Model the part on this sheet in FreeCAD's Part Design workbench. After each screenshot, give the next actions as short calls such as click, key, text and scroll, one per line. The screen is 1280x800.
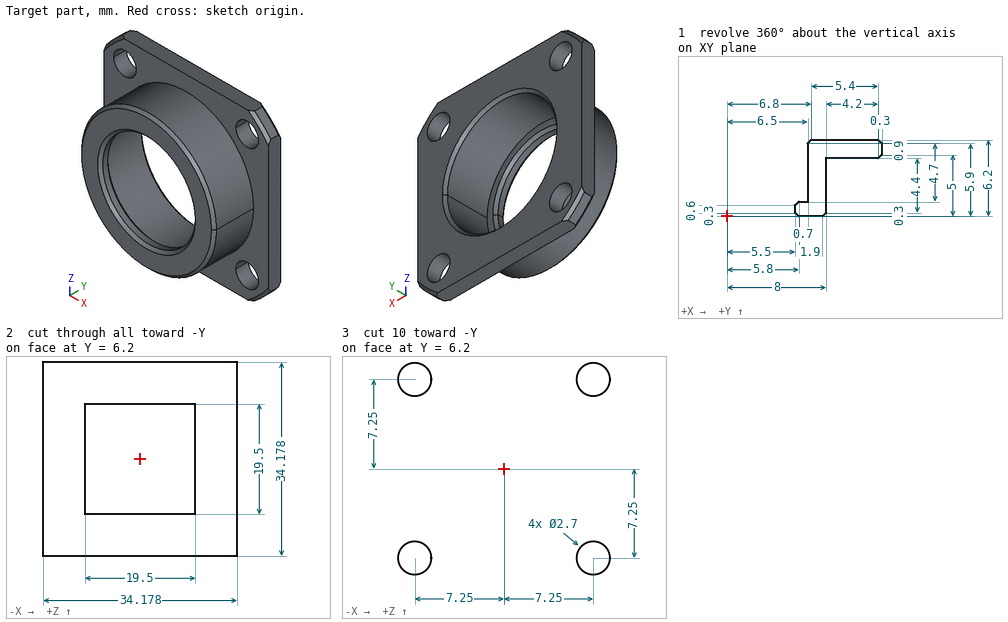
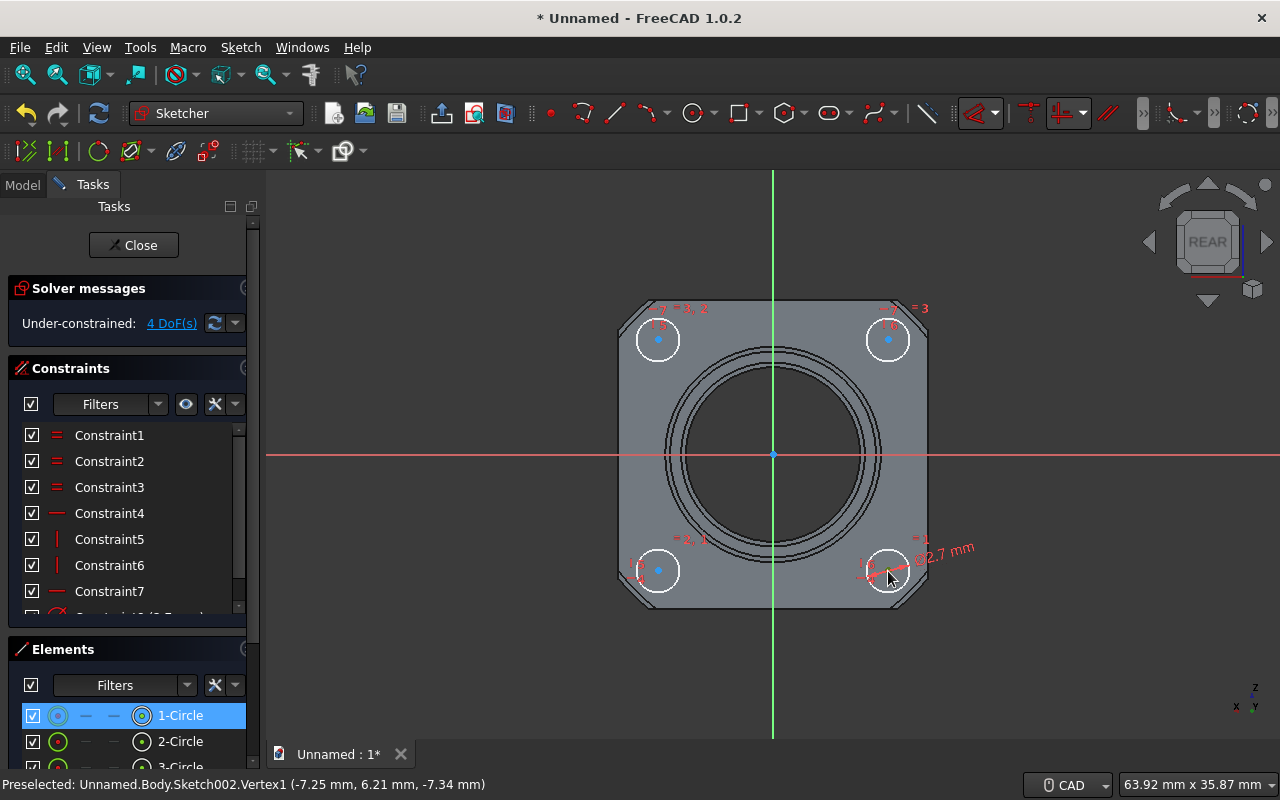
click(998, 114)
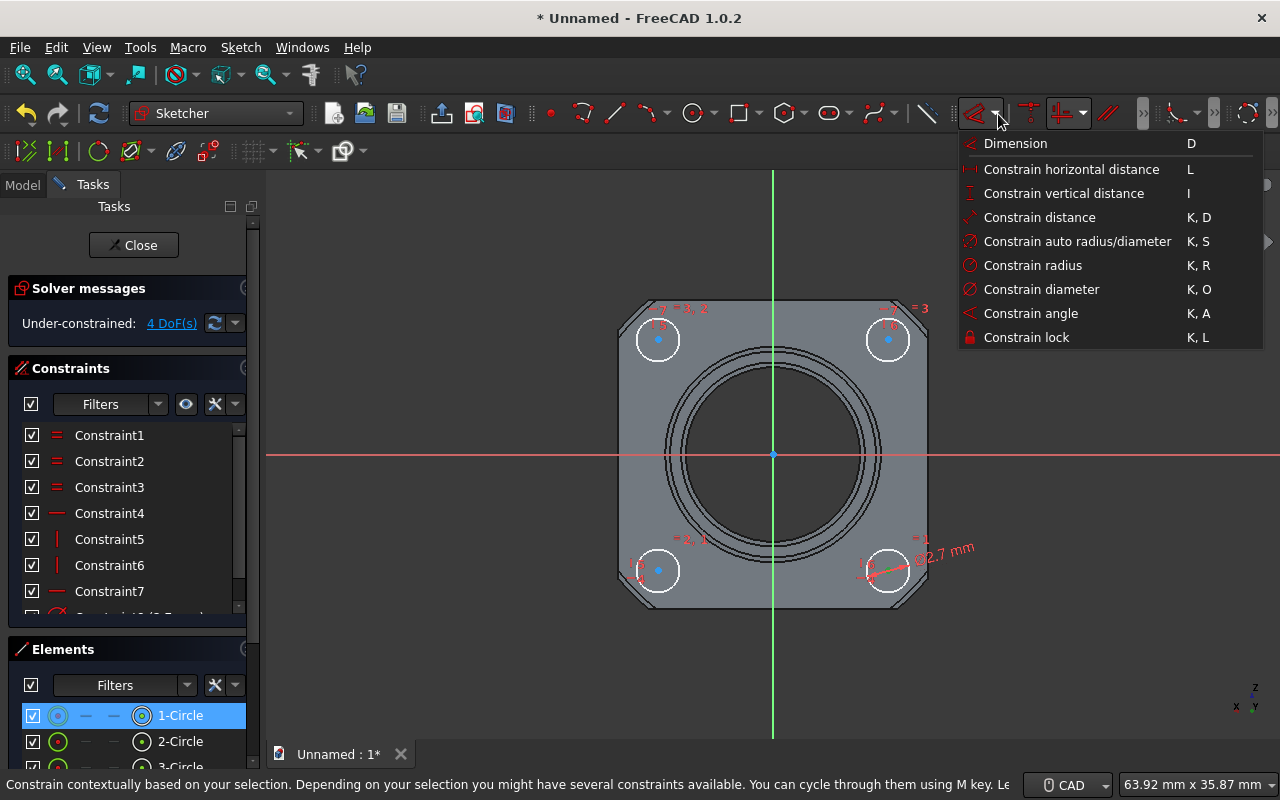
click(1111, 169)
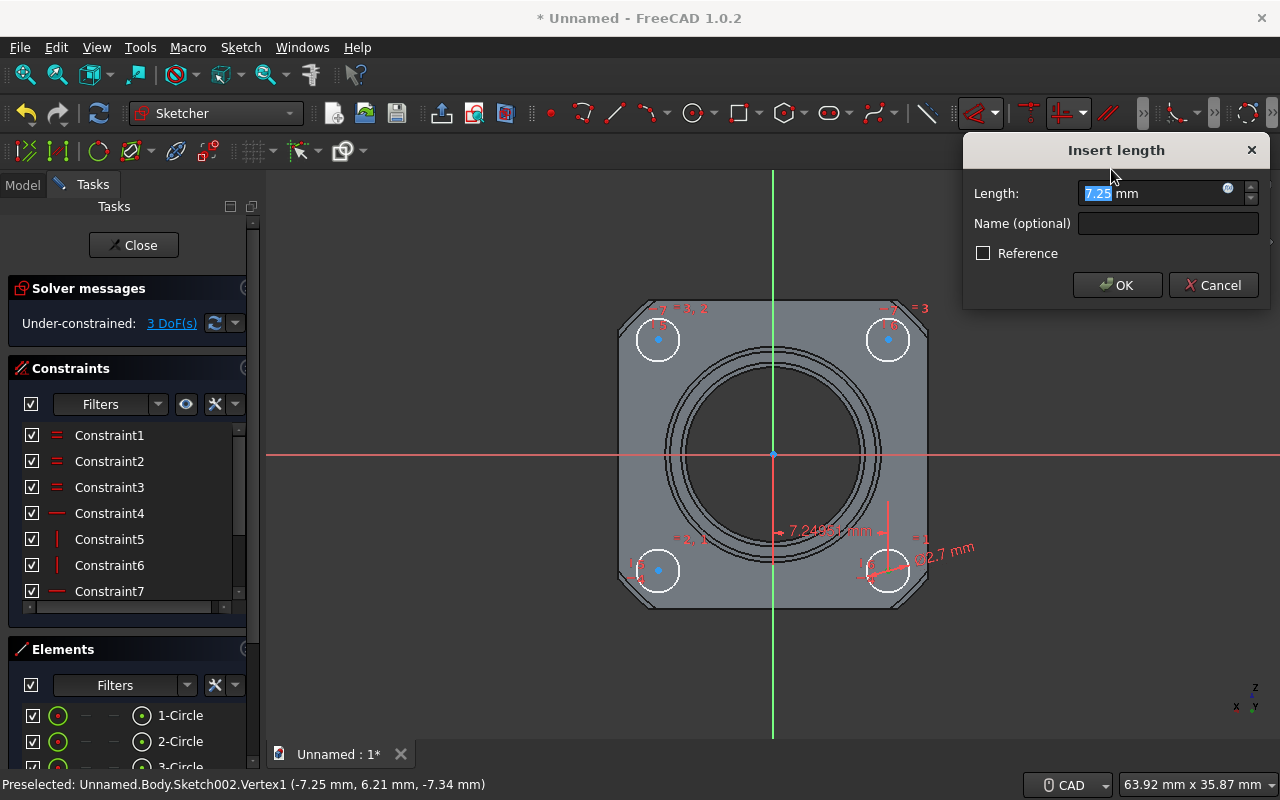
text(7.25)
key(Return)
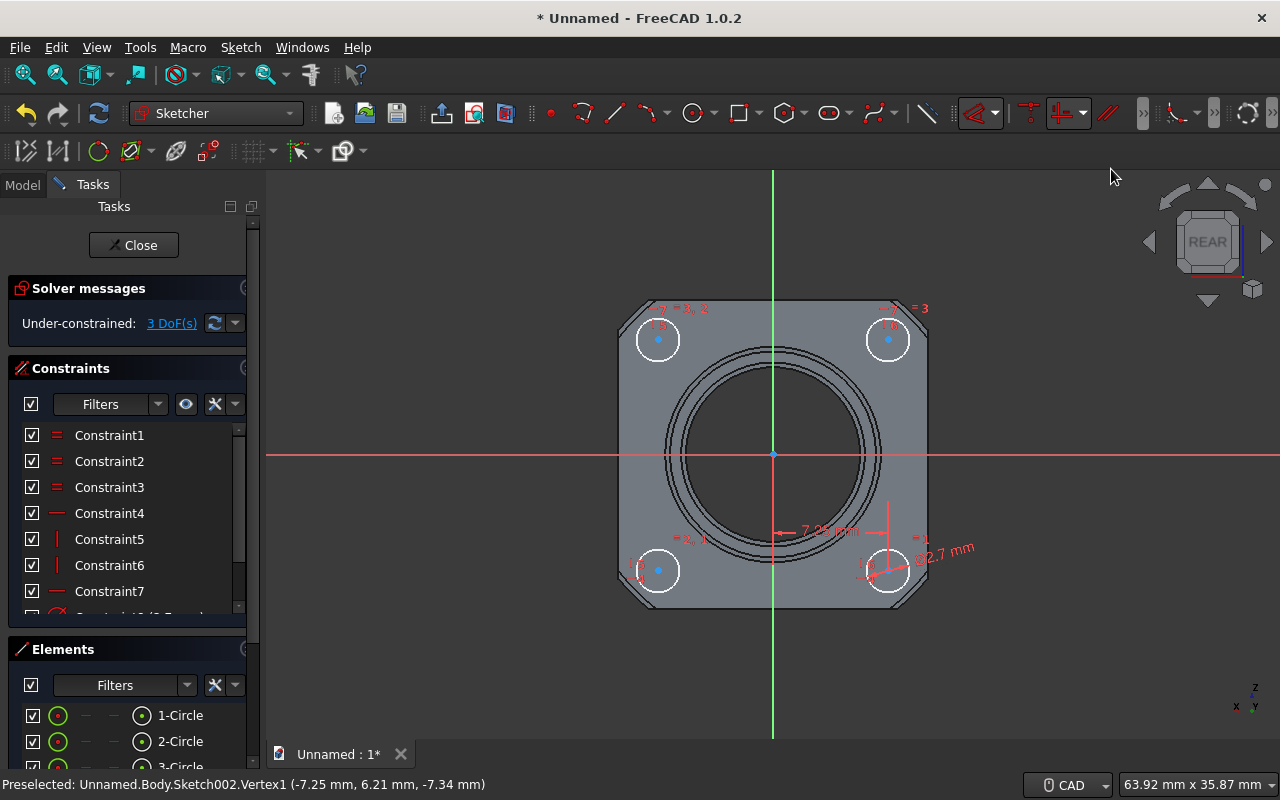
click(888, 571)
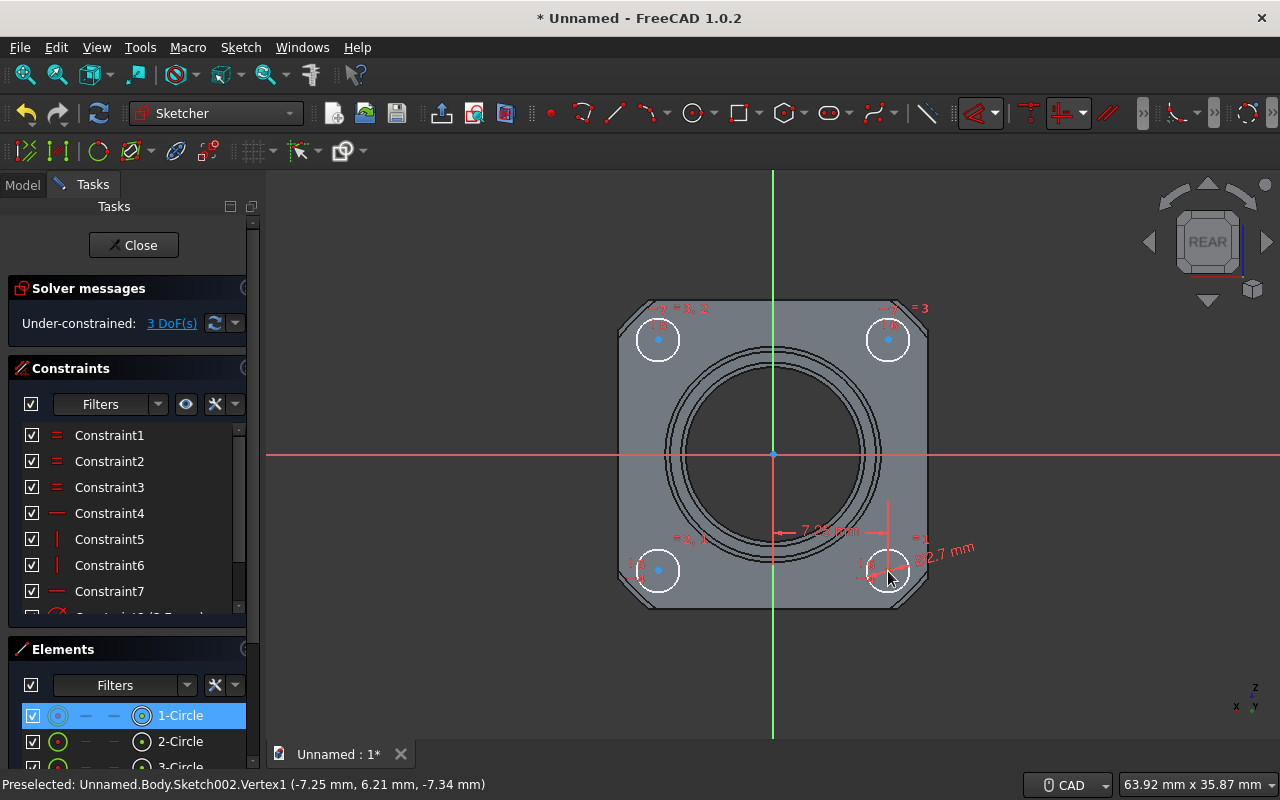
key(i)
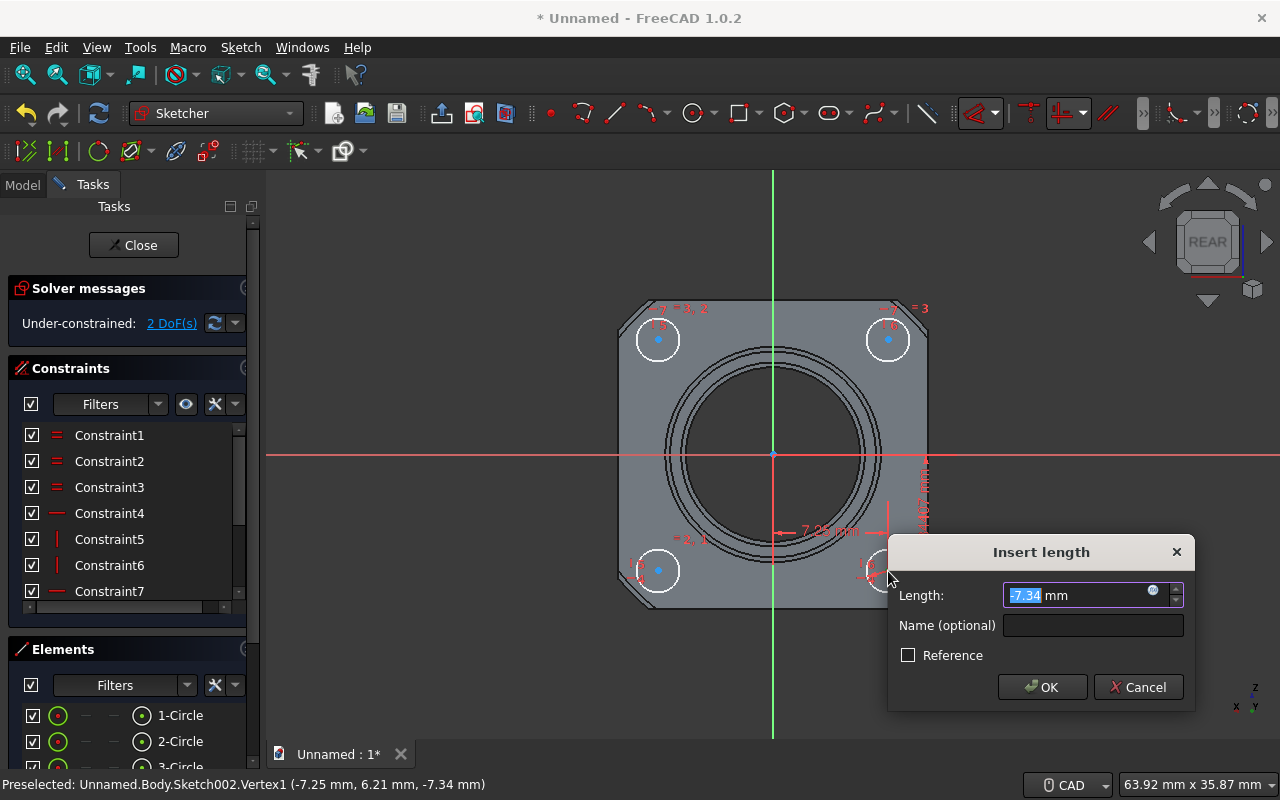
text(-7.25)
key(Return)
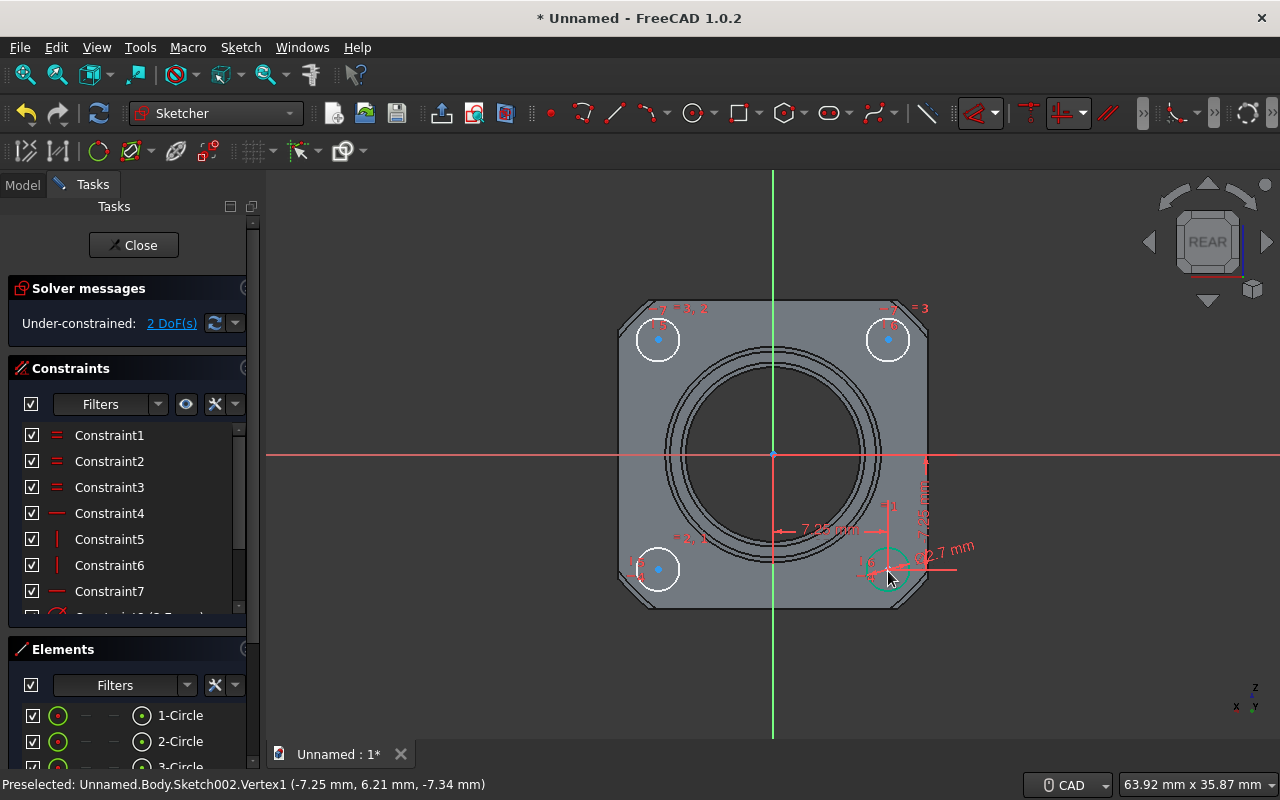
click(658, 570)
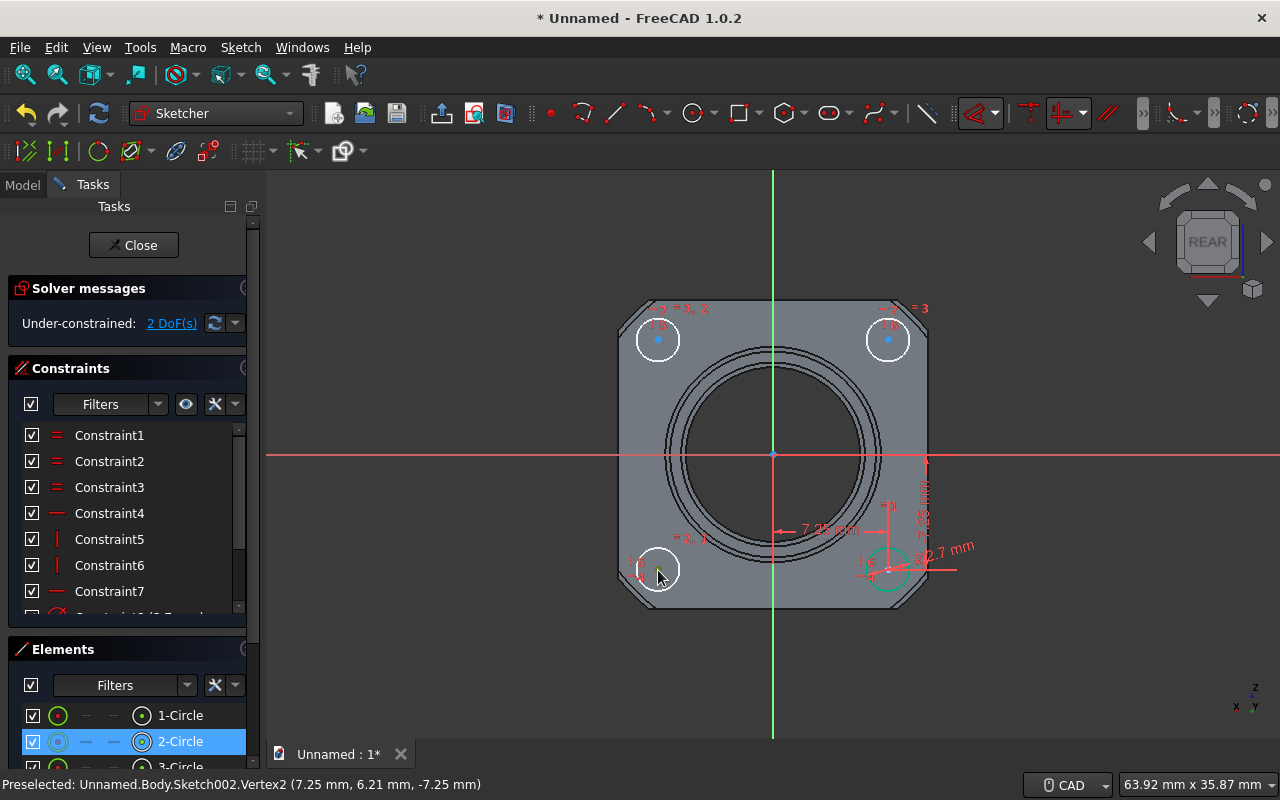
key(l)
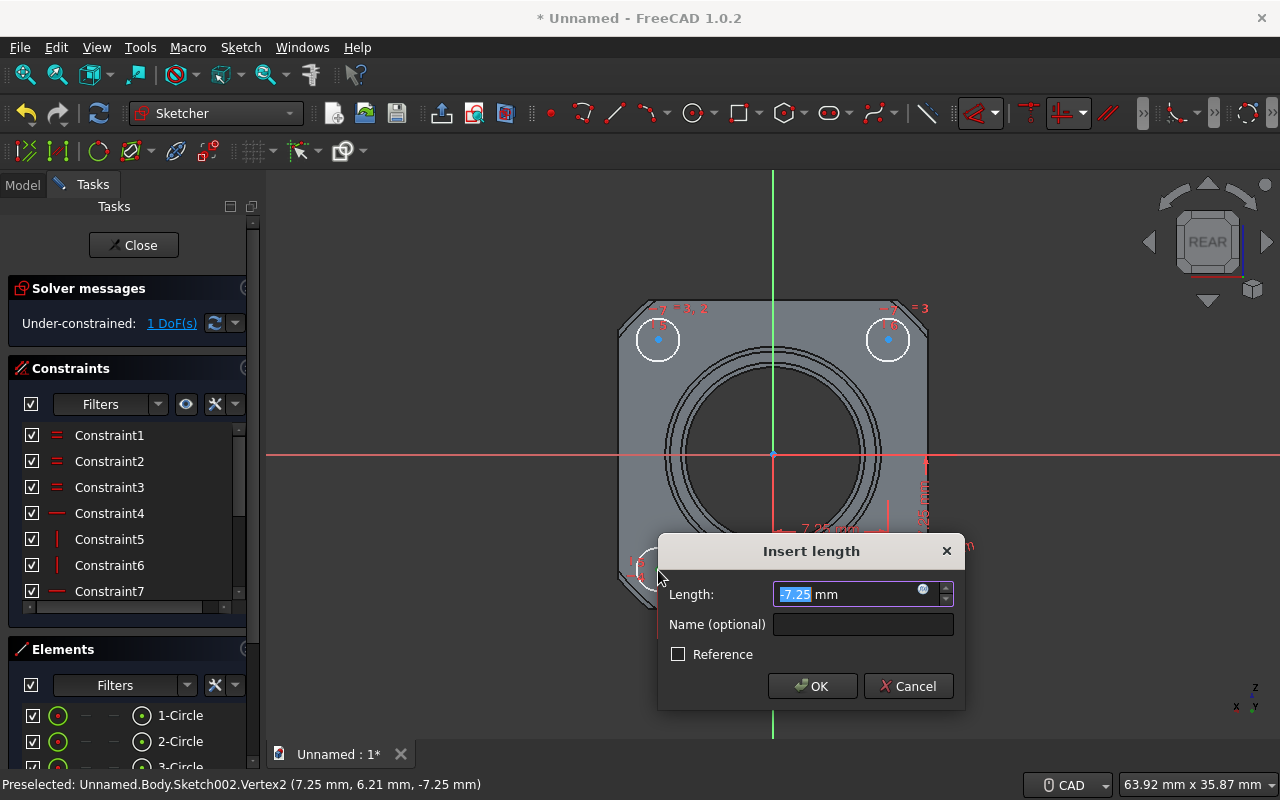
text(-7.25)
key(Return)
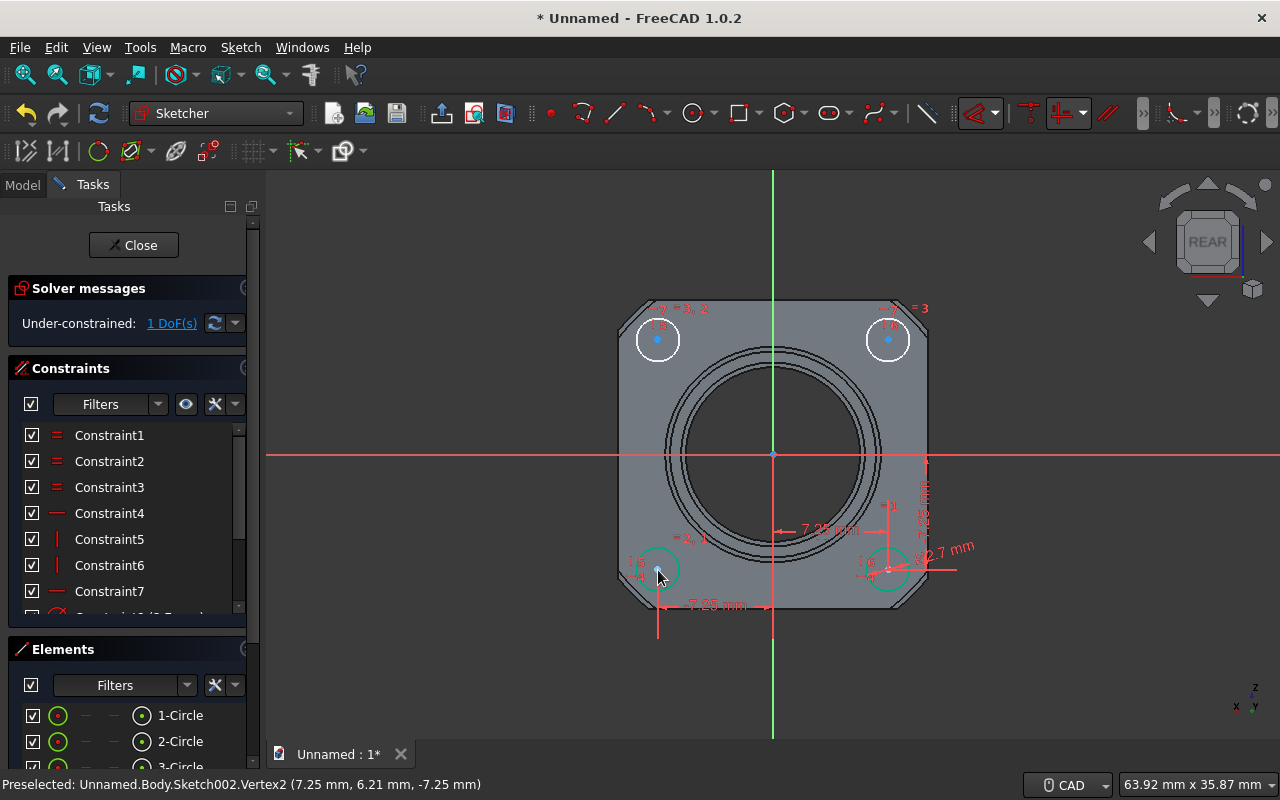
click(658, 340)